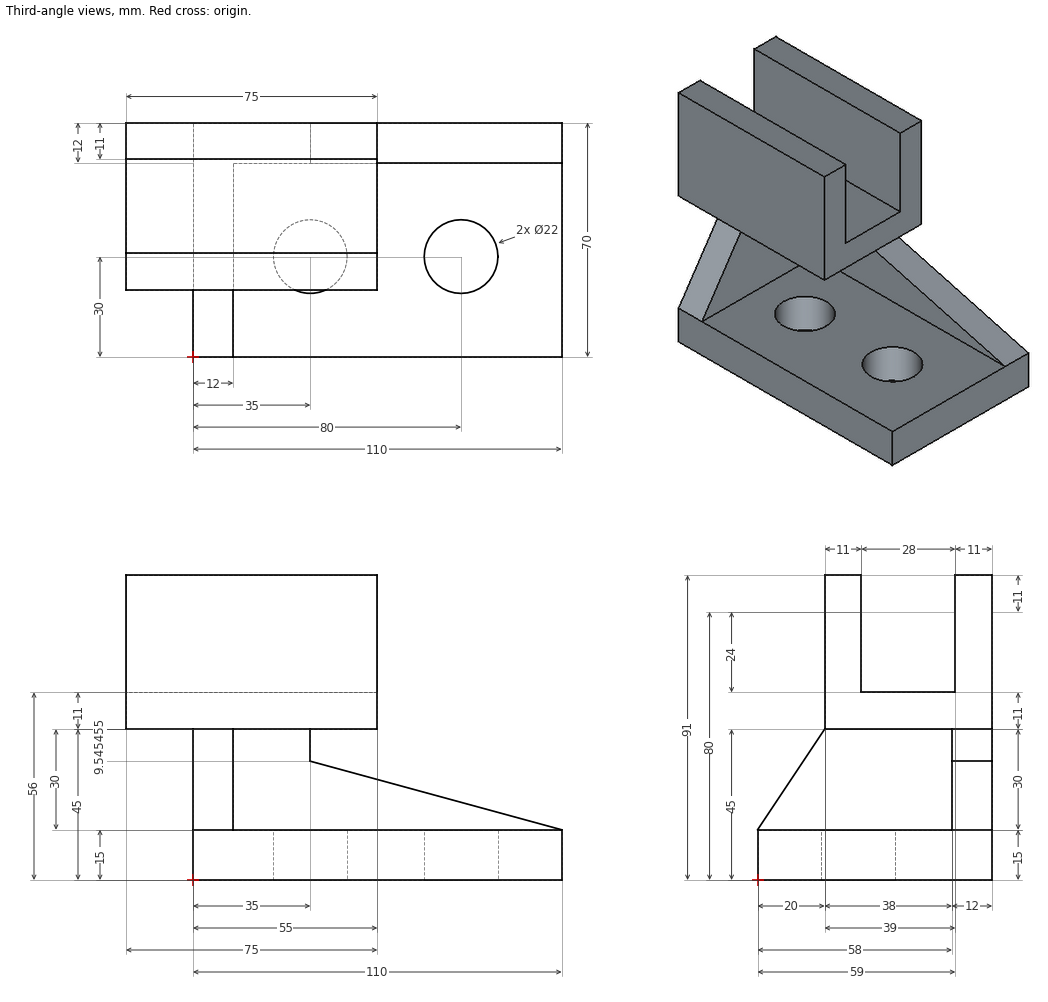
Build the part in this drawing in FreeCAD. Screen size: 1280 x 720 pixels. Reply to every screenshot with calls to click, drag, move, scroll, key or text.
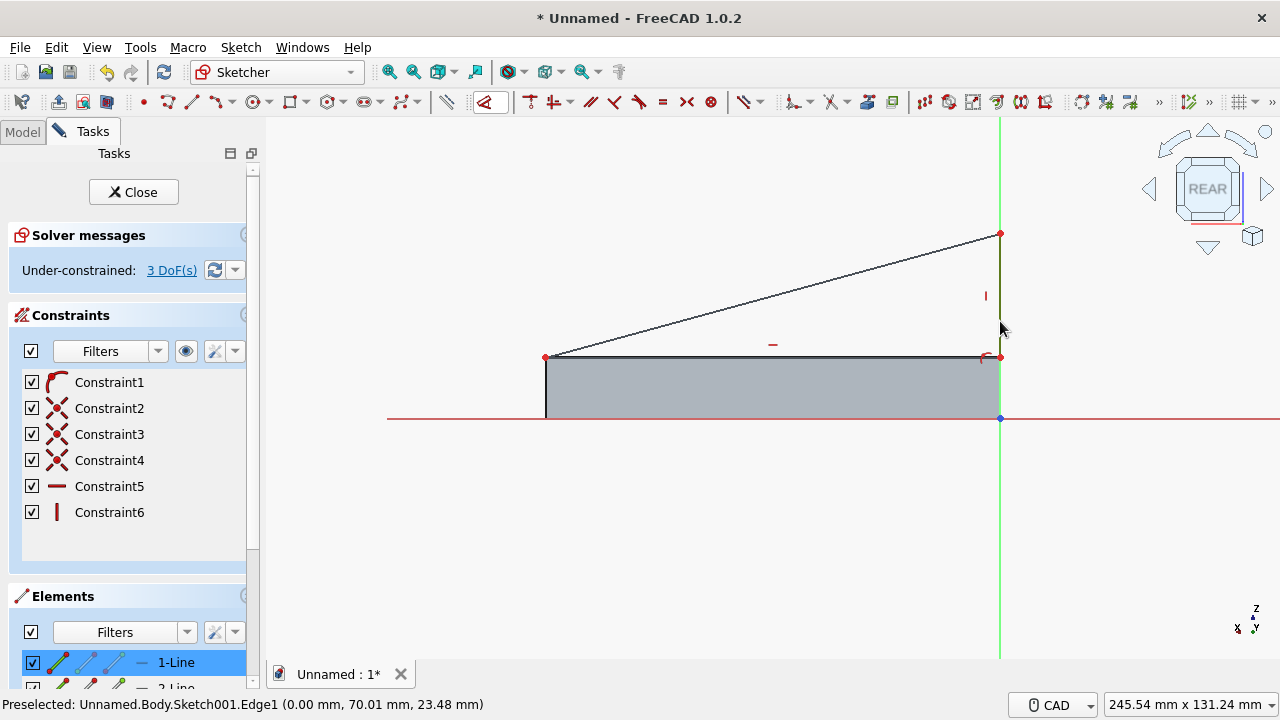
key(i)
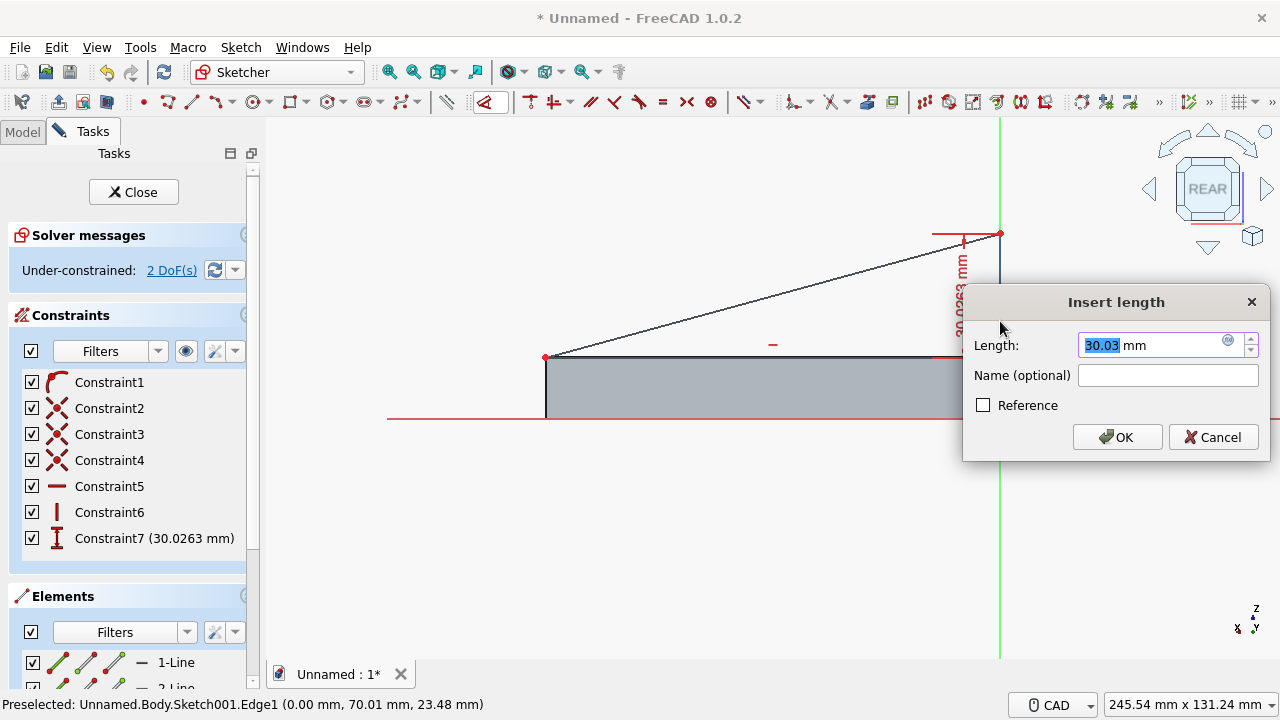
text(30)
key(Return)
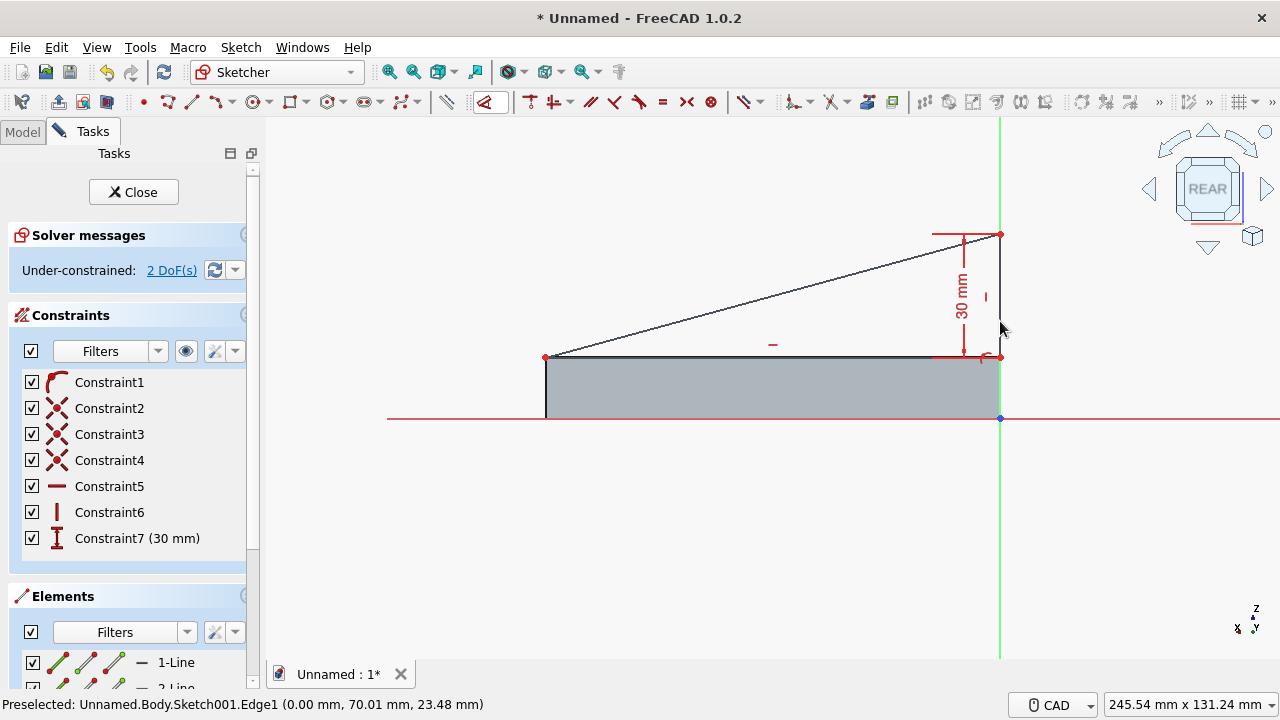
click(682, 358)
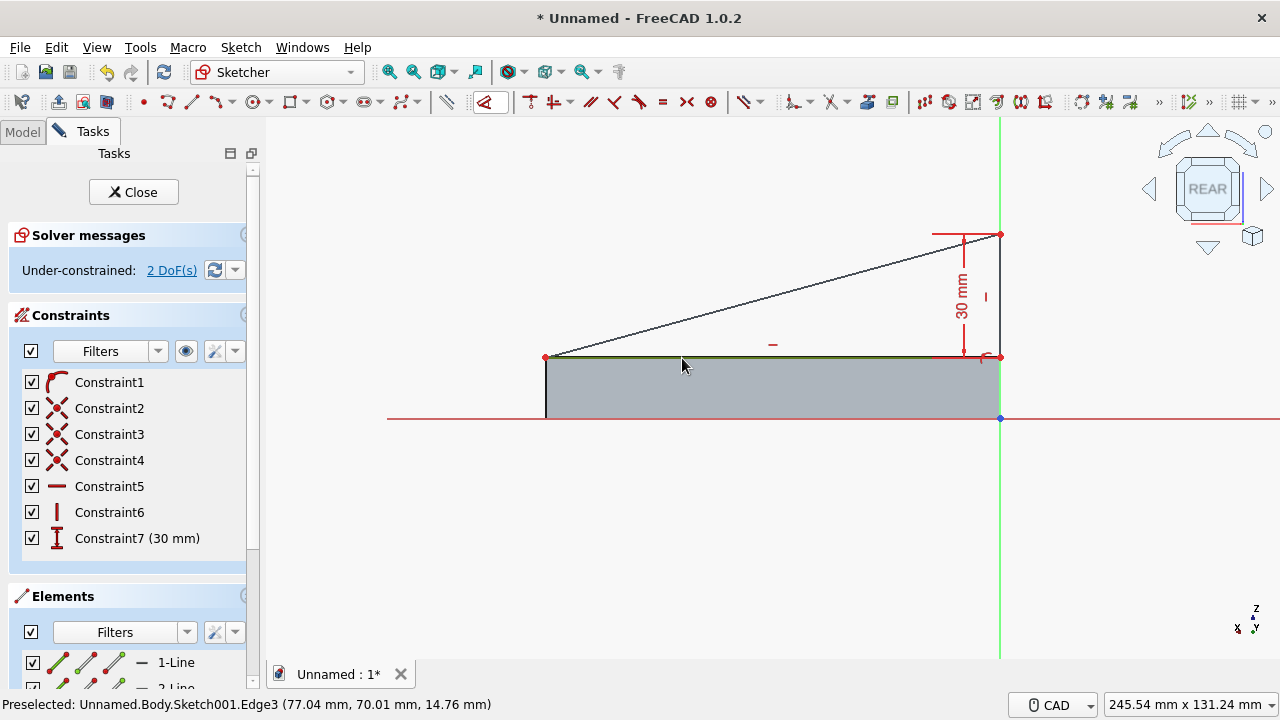
key(l)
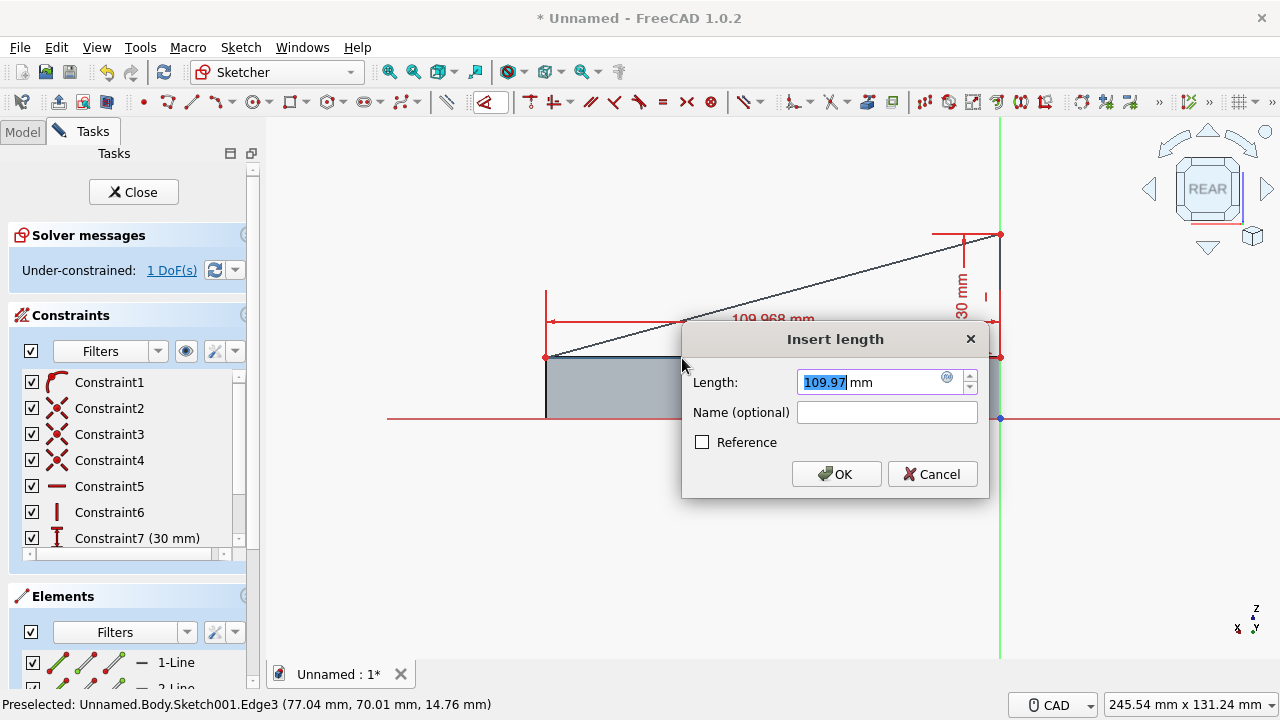
text(110)
key(Return)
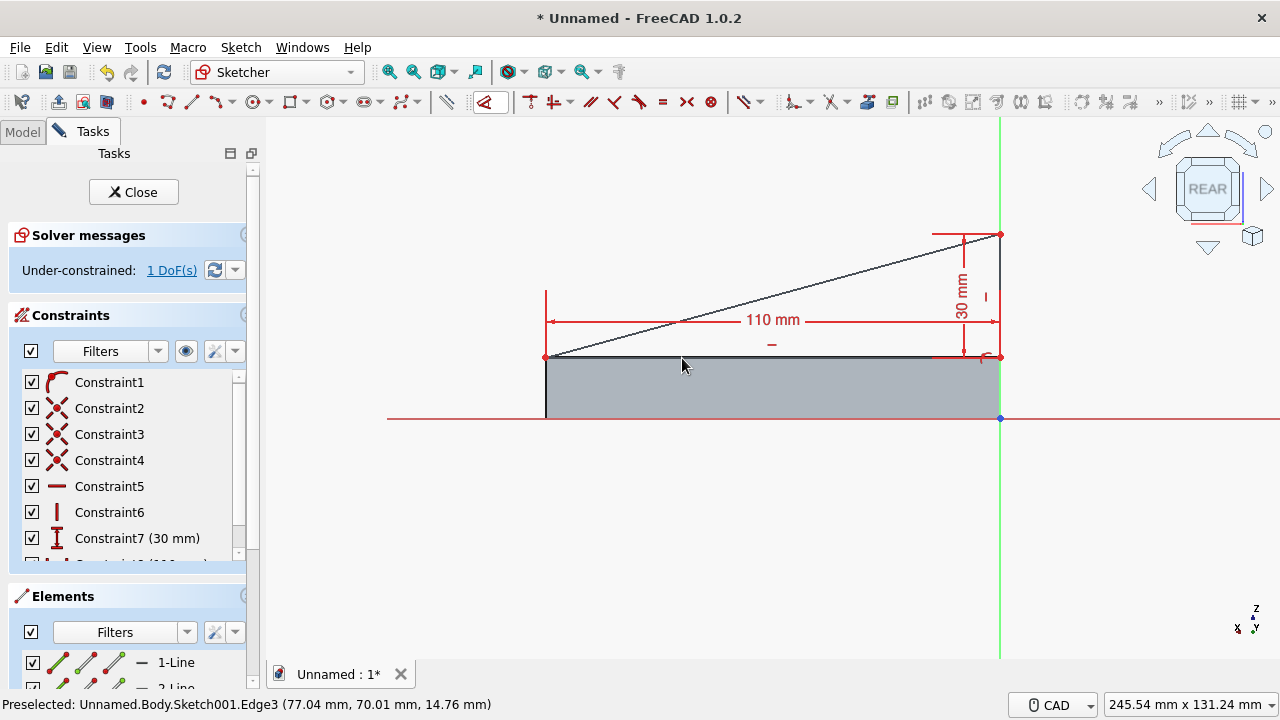
click(1000, 358)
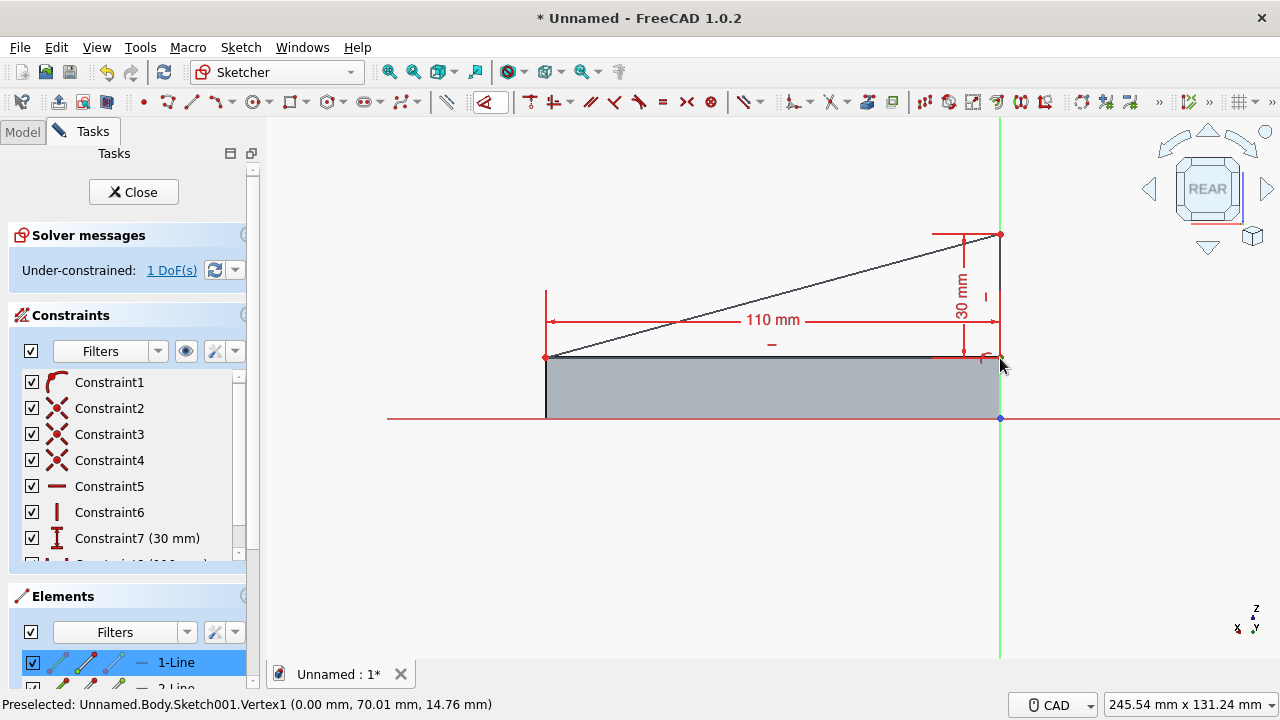
key(i)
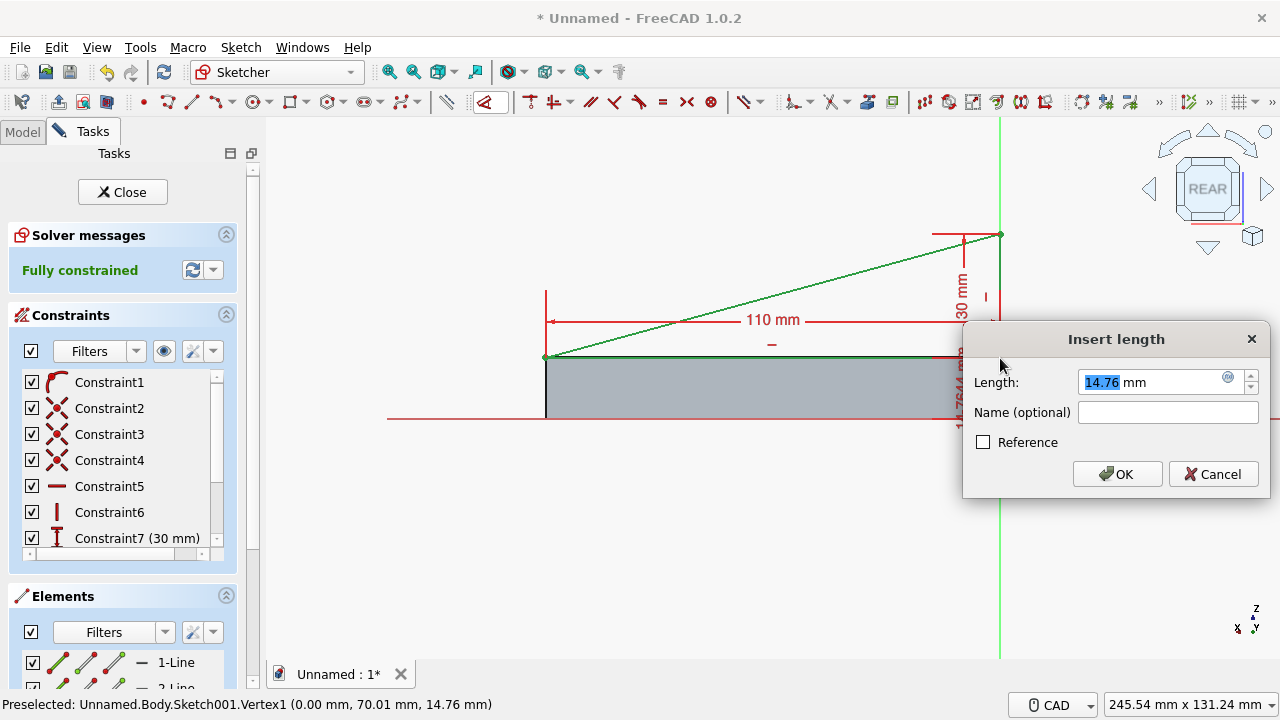
text(15)
key(Return)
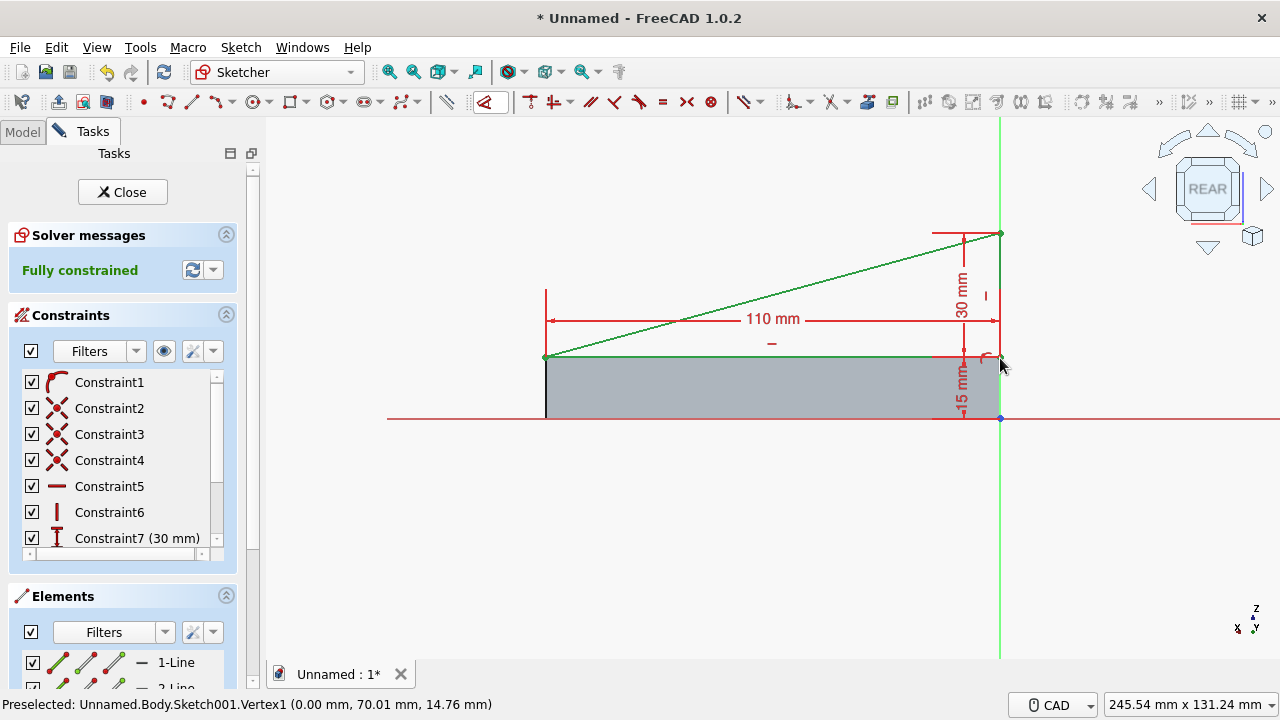
click(123, 192)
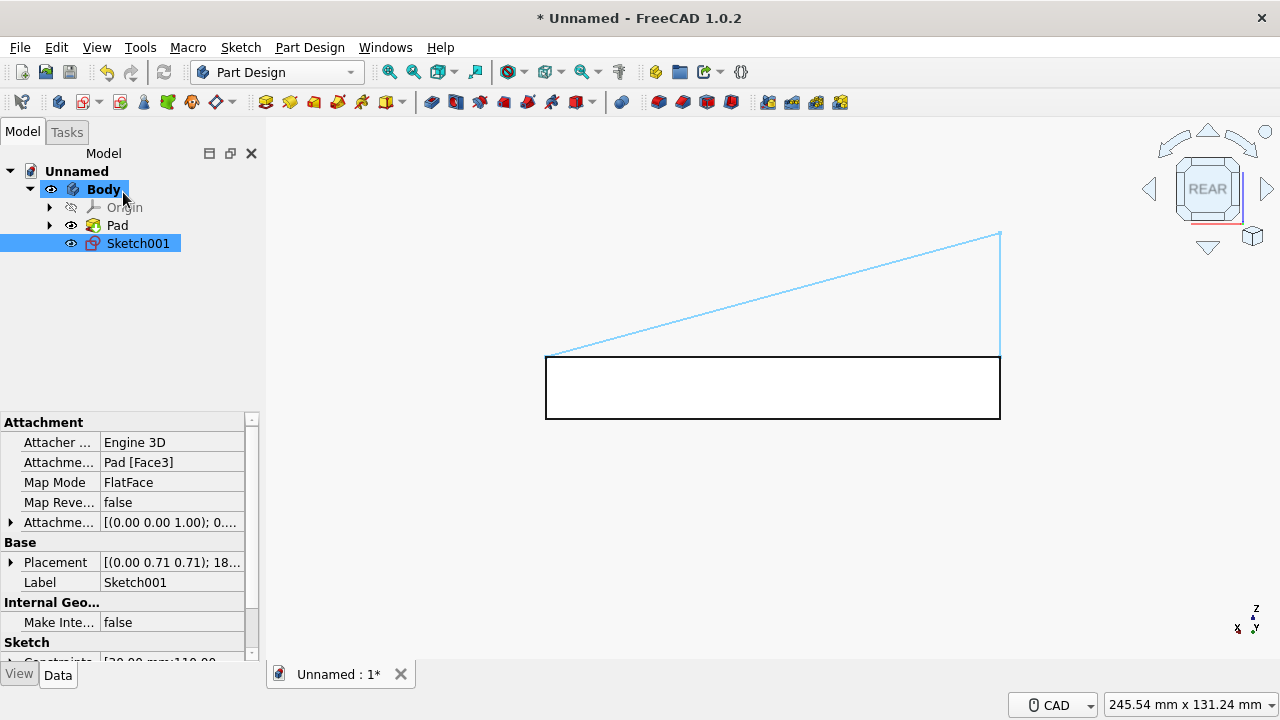
click(266, 102)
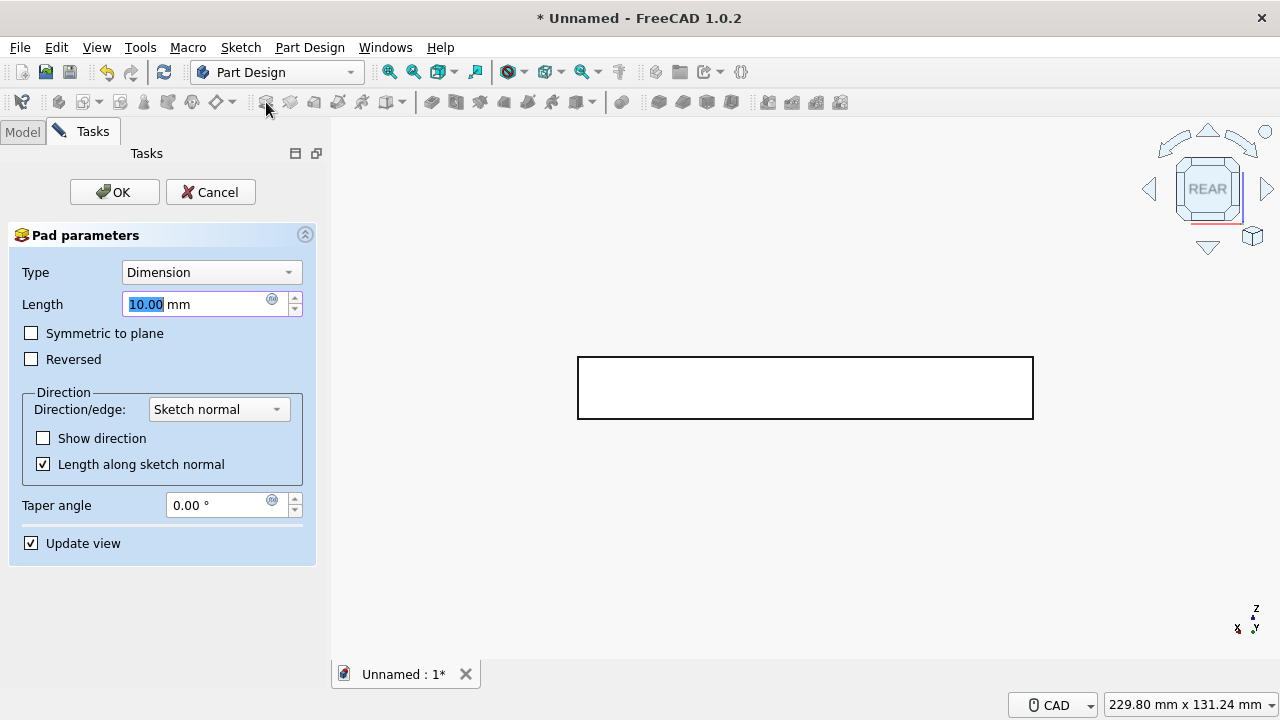
text(12)
key(Tab)